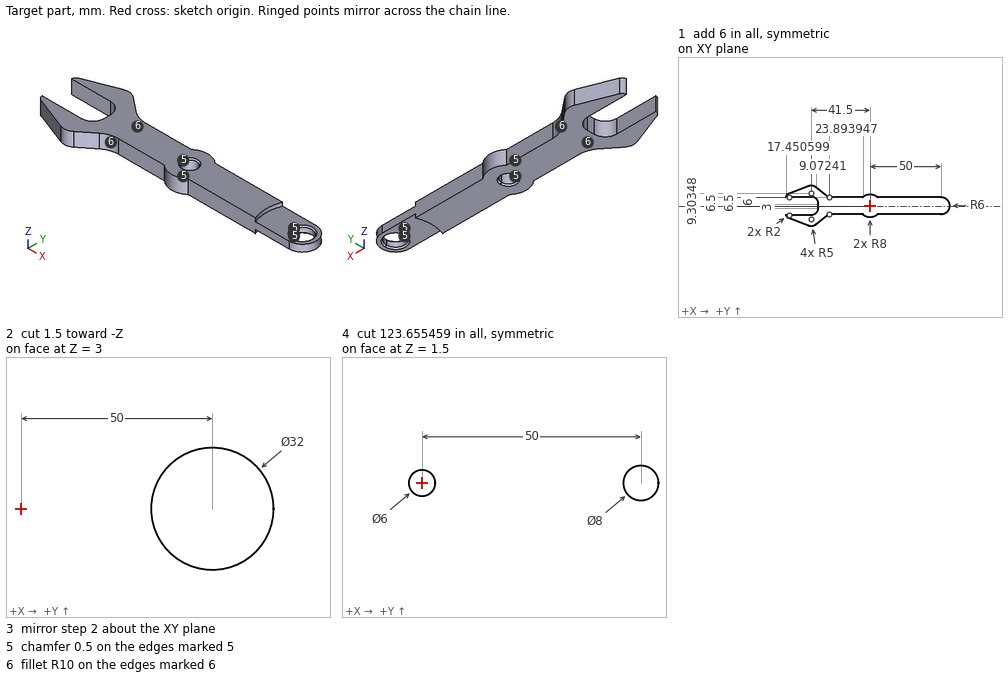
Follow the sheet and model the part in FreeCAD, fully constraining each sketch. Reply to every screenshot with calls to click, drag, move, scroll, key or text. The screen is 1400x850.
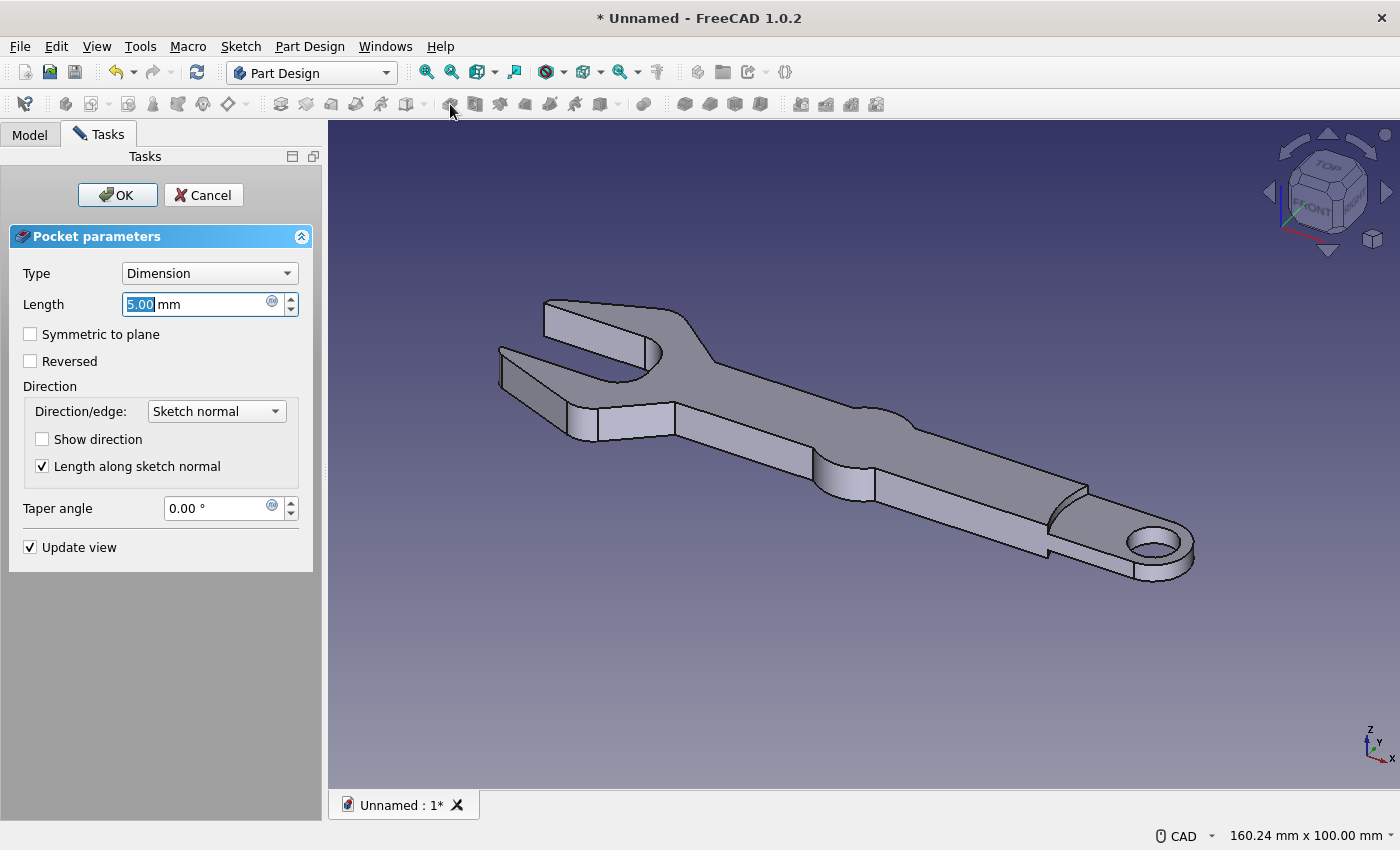
text(123.655459)
key(Tab)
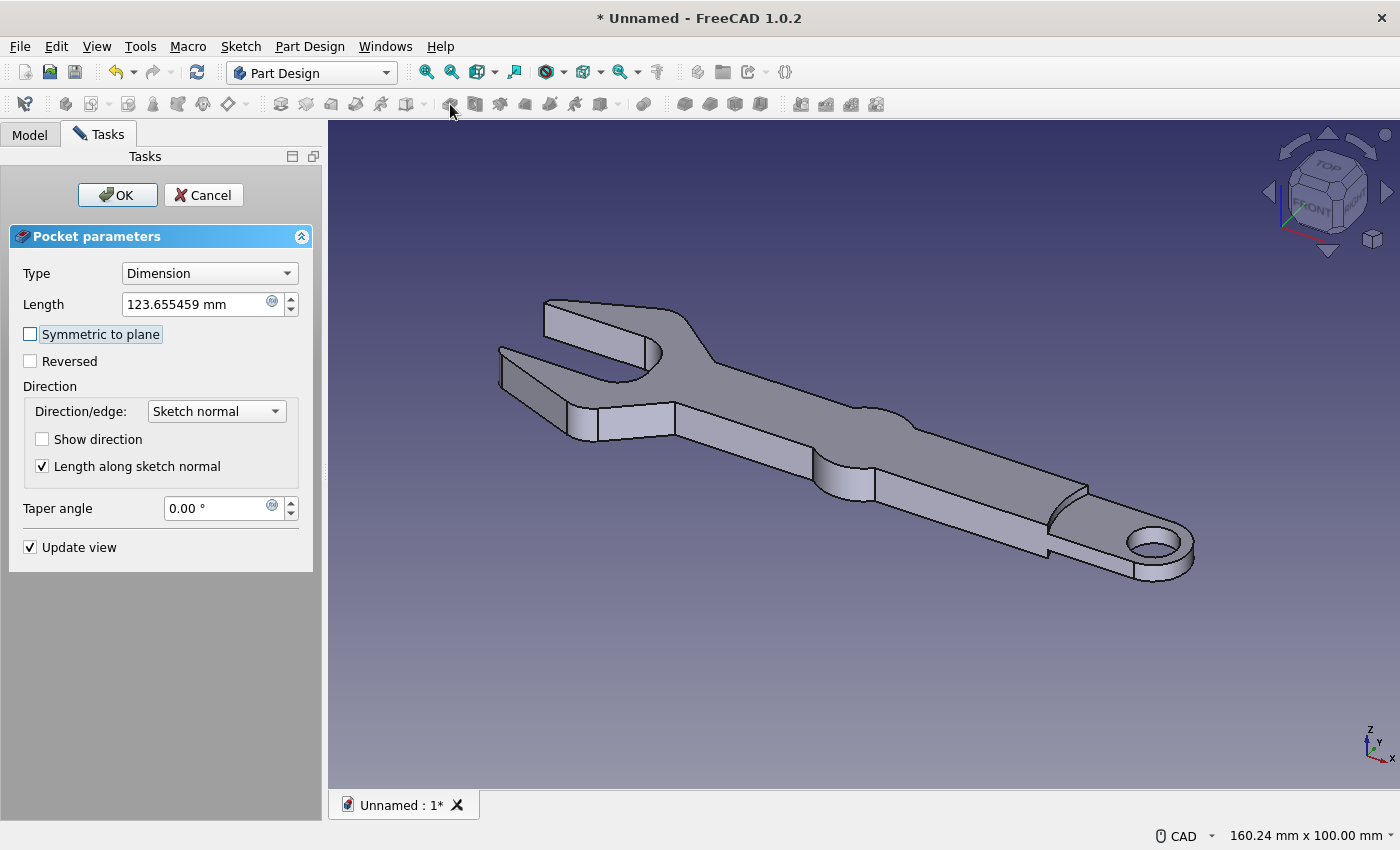
click(31, 334)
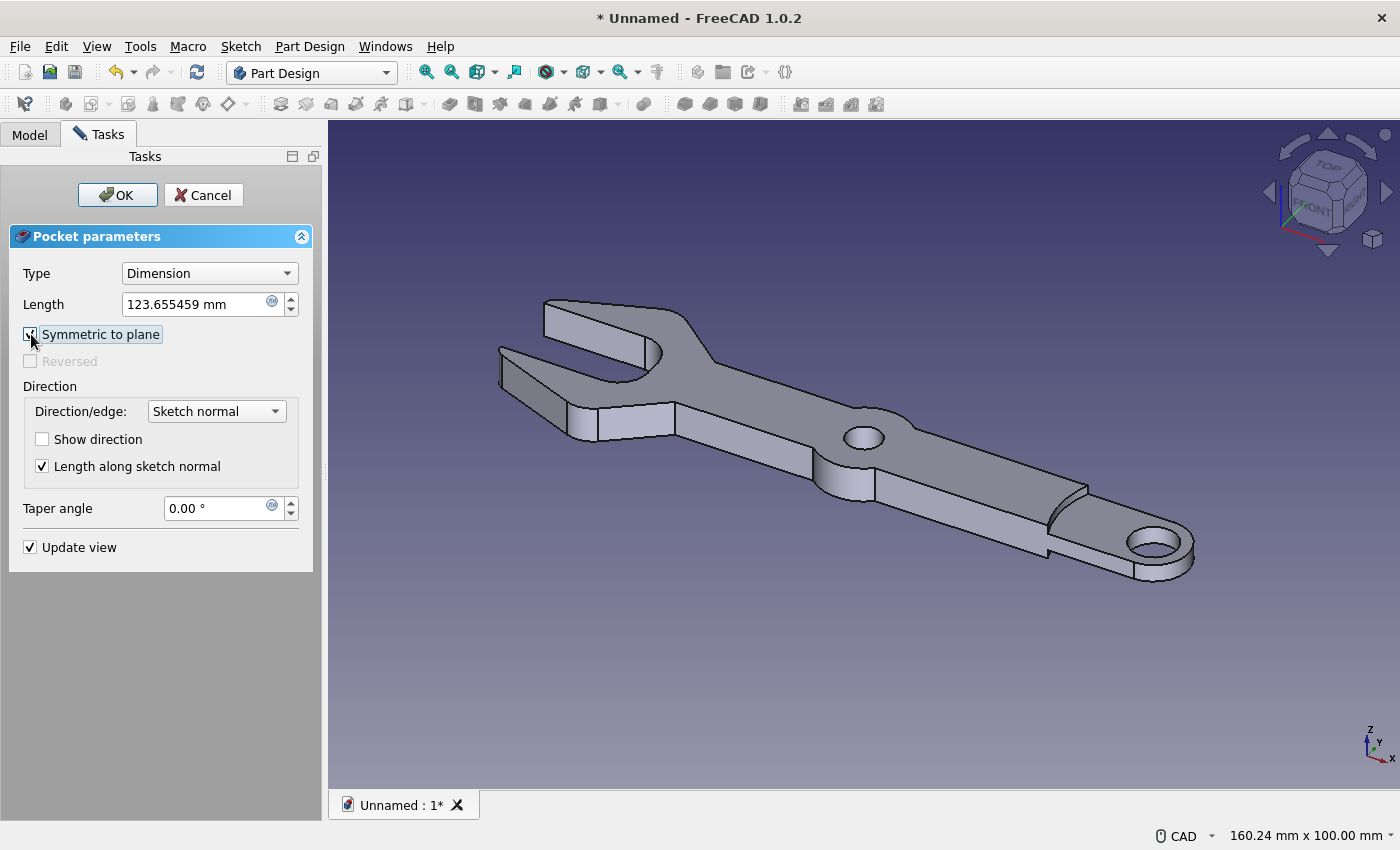
click(118, 195)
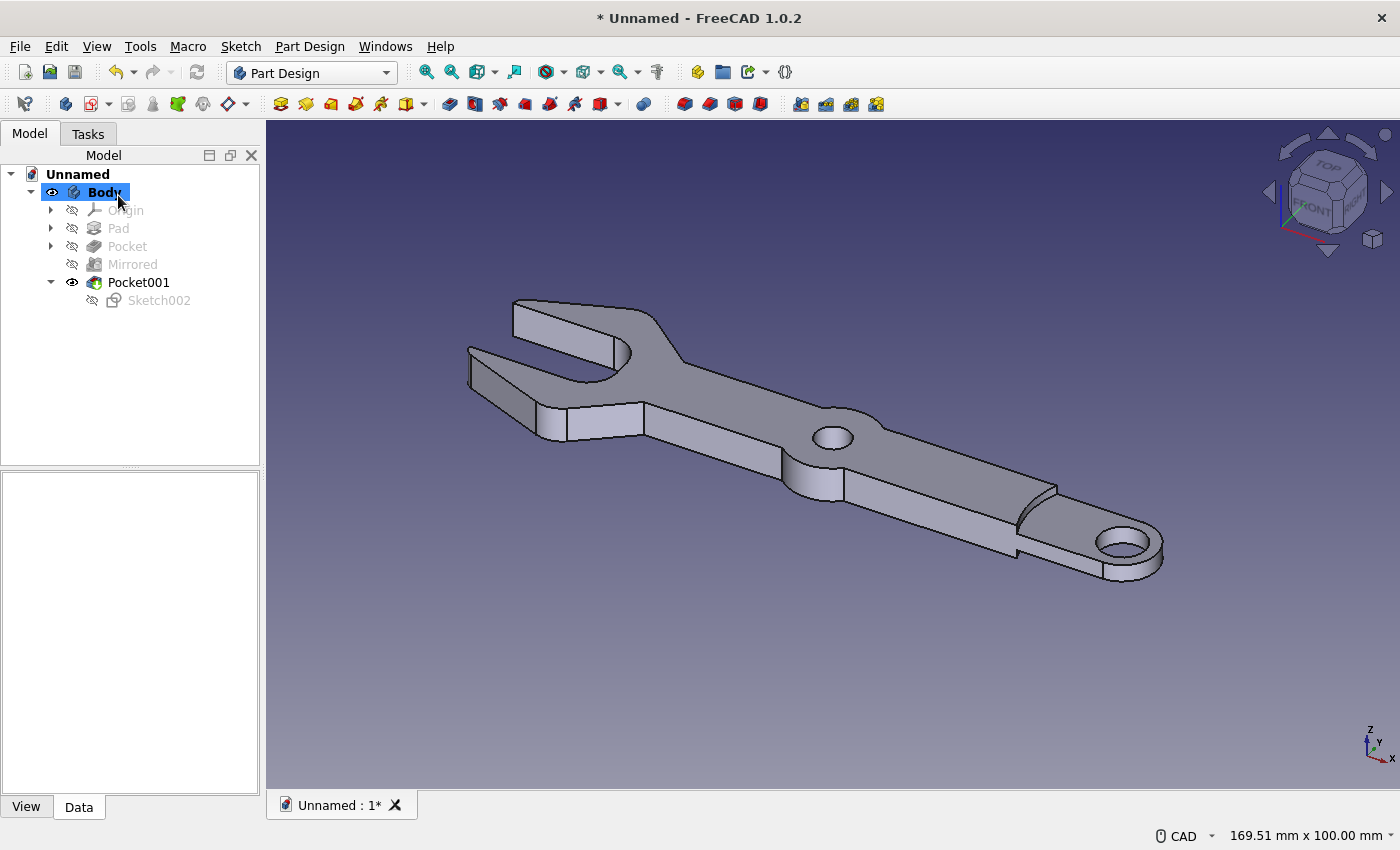
click(1100, 534)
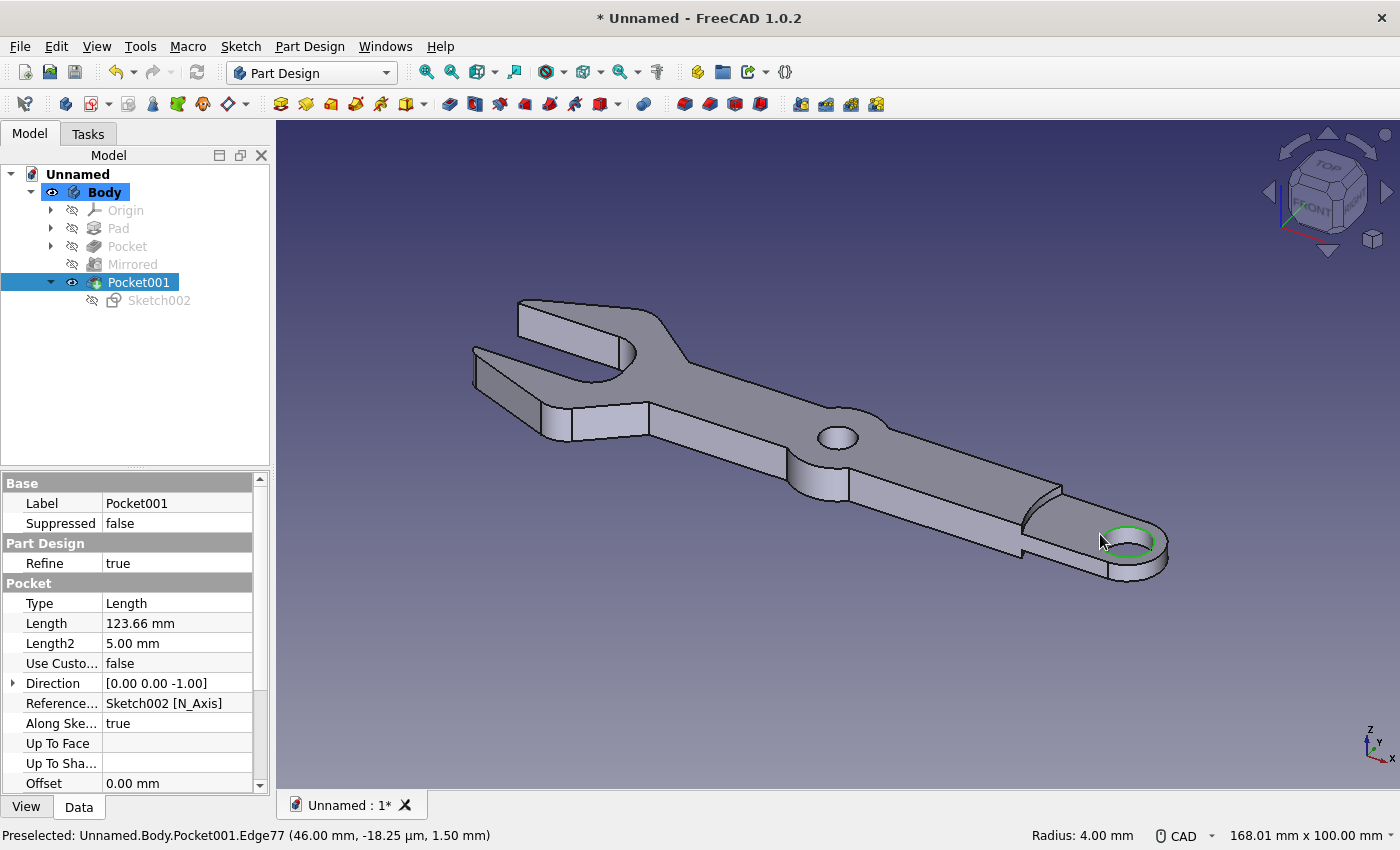
click(821, 431, ctrl)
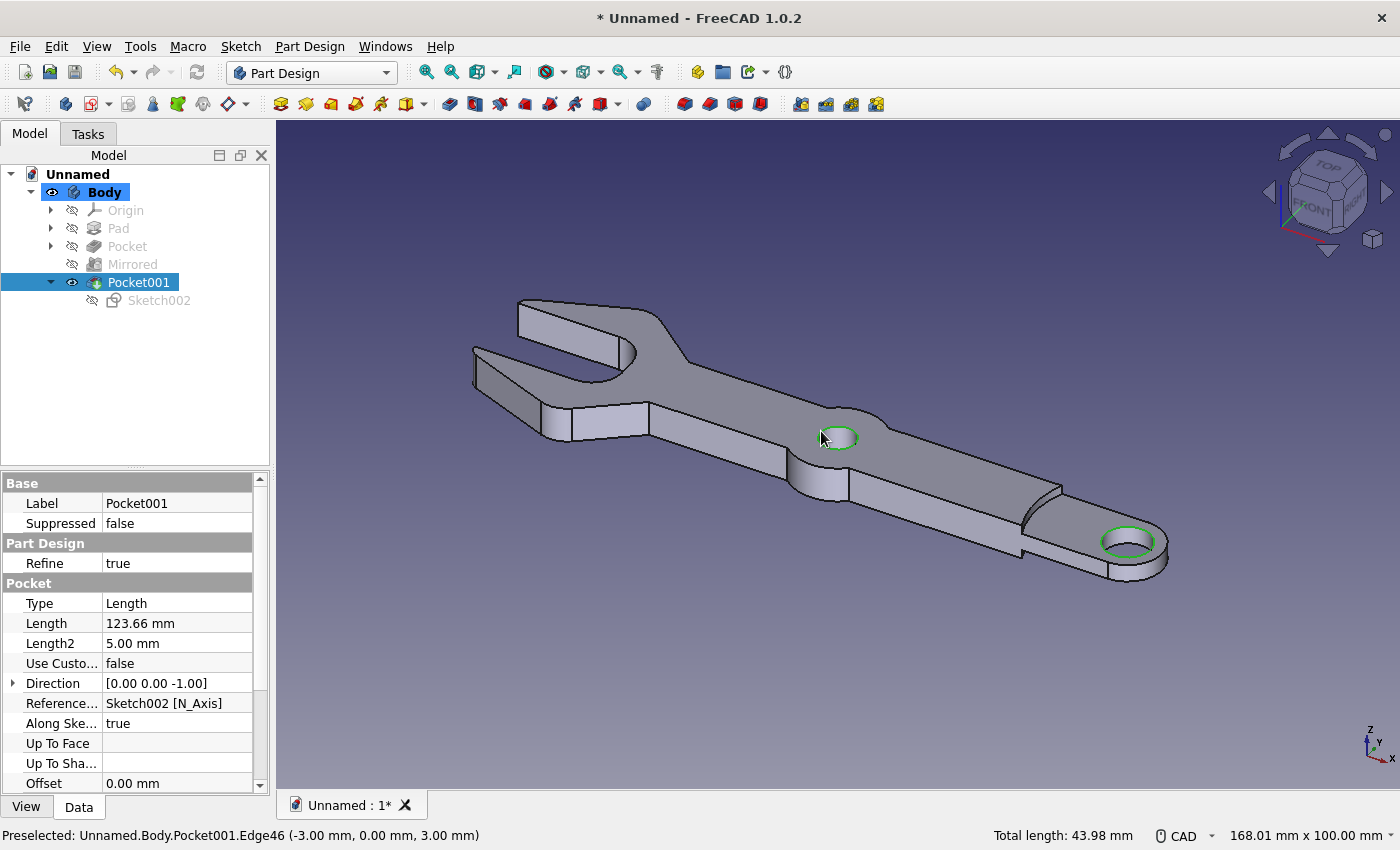
key(0)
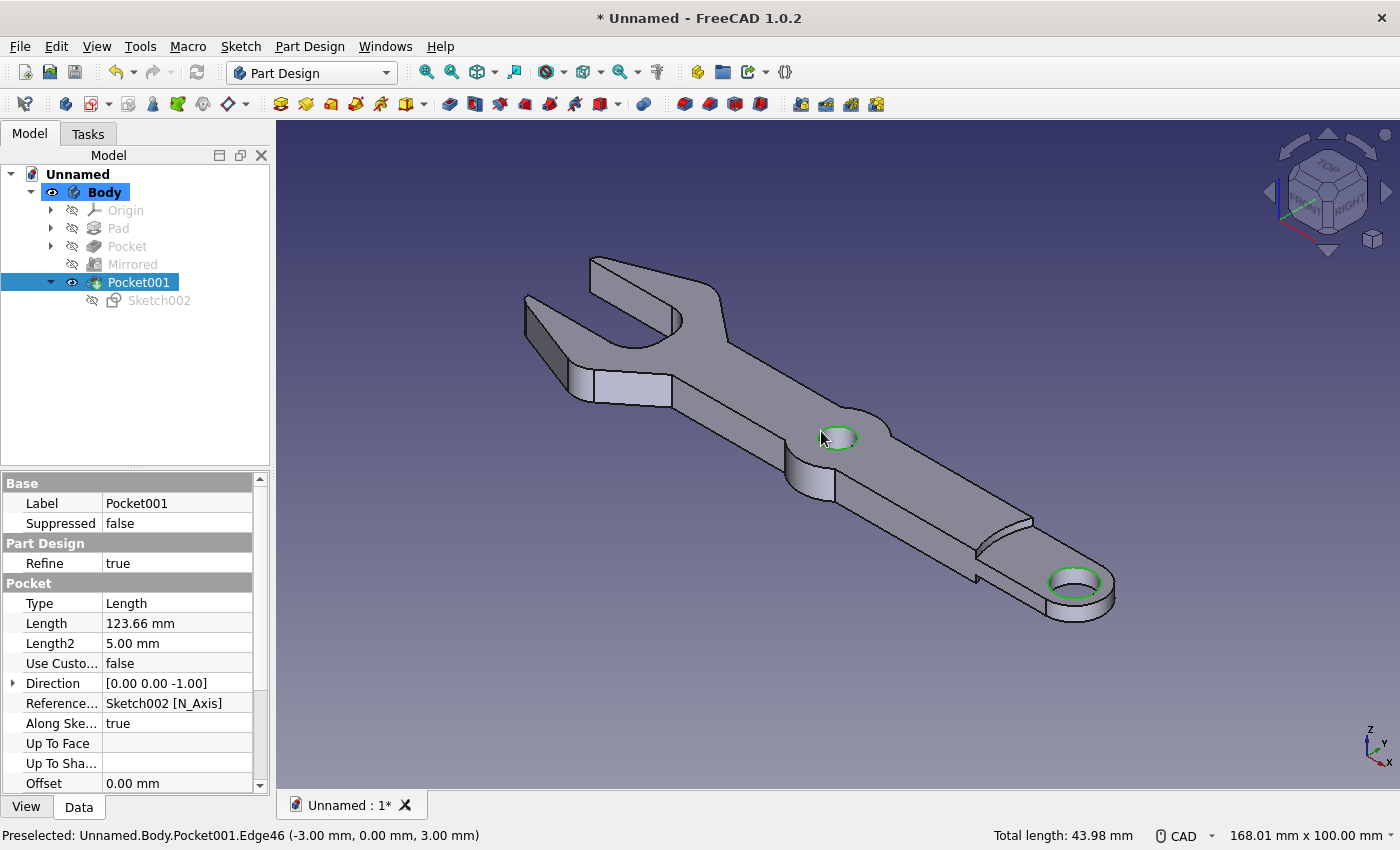
key(2)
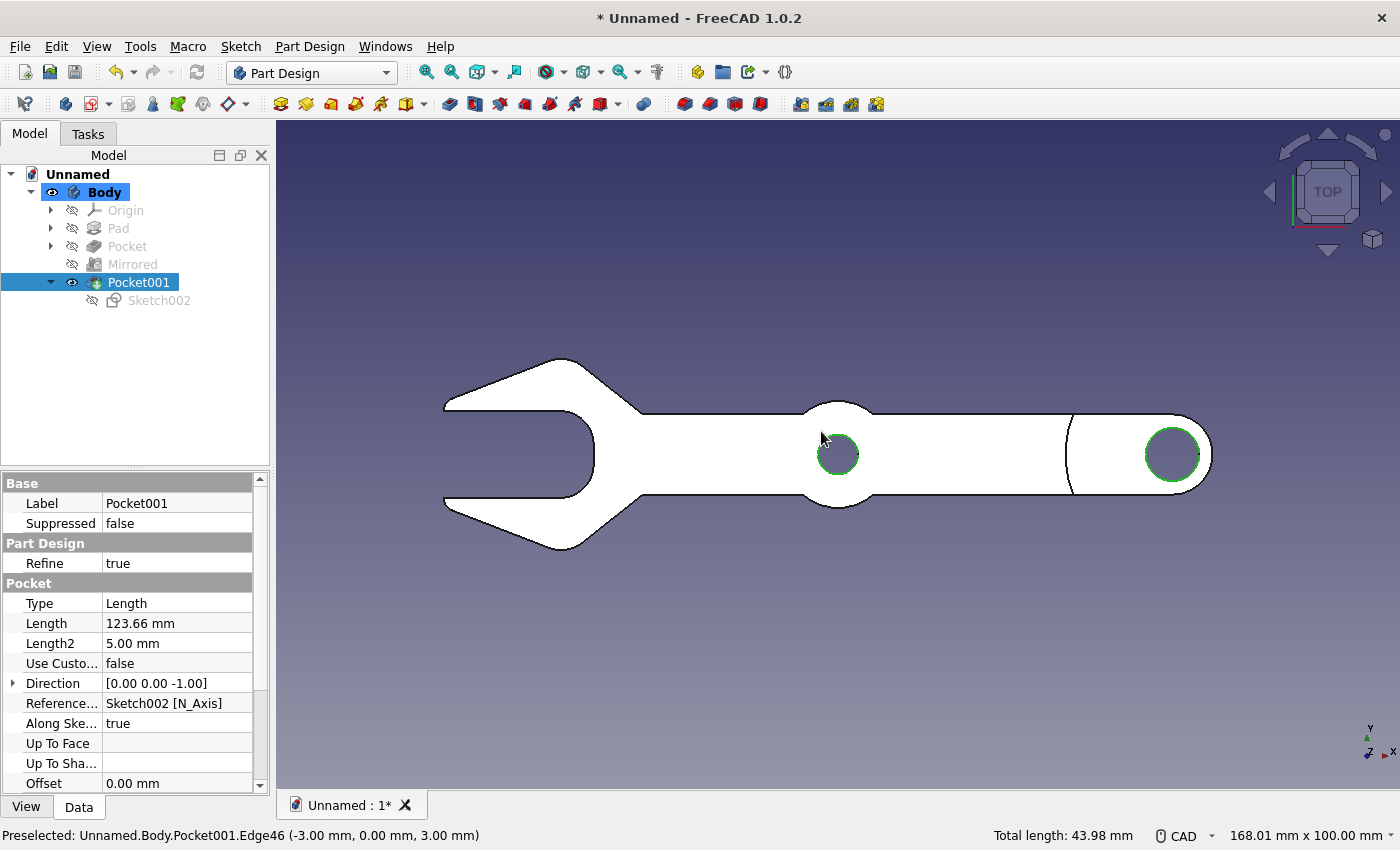
key(1)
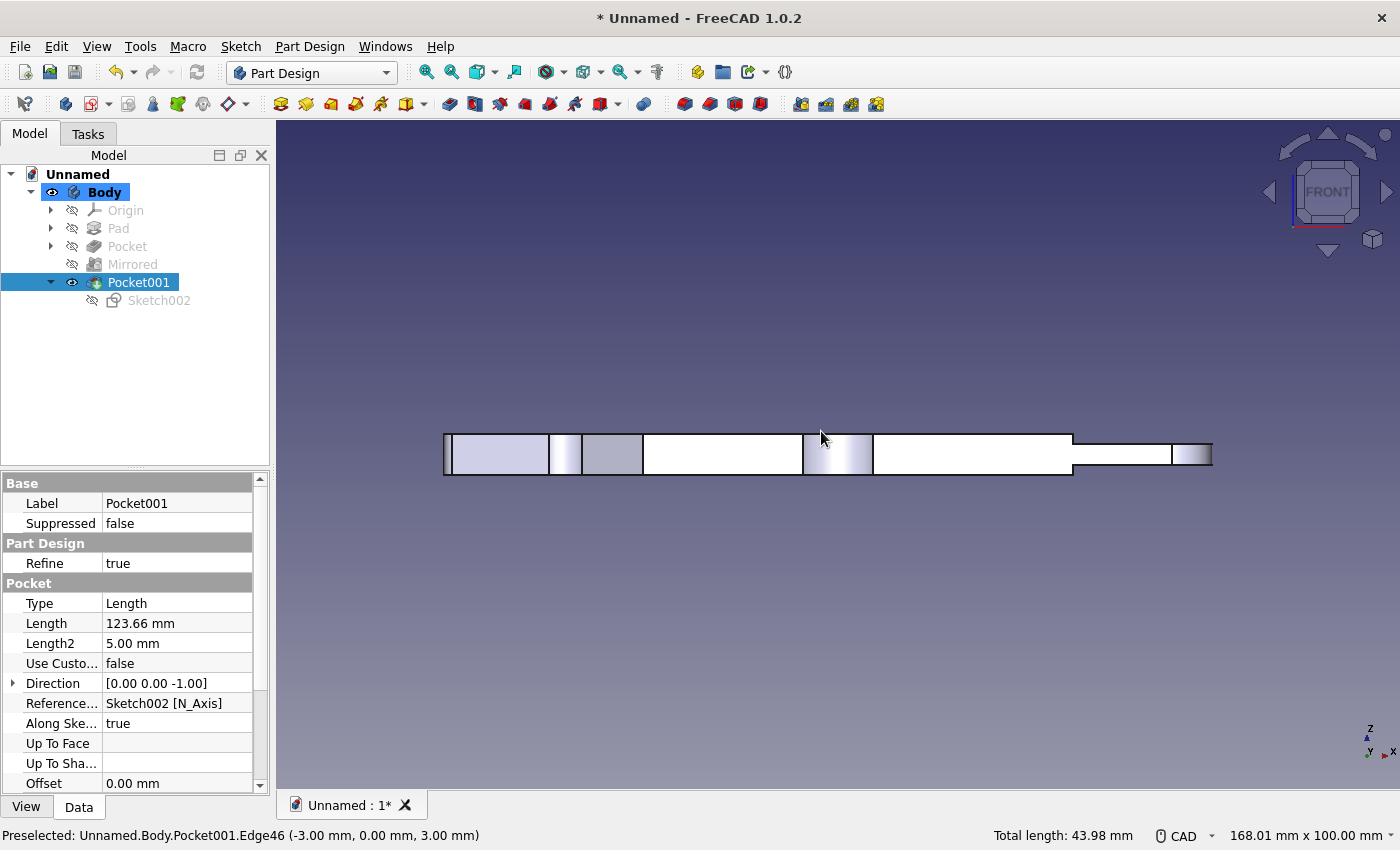
key(3)